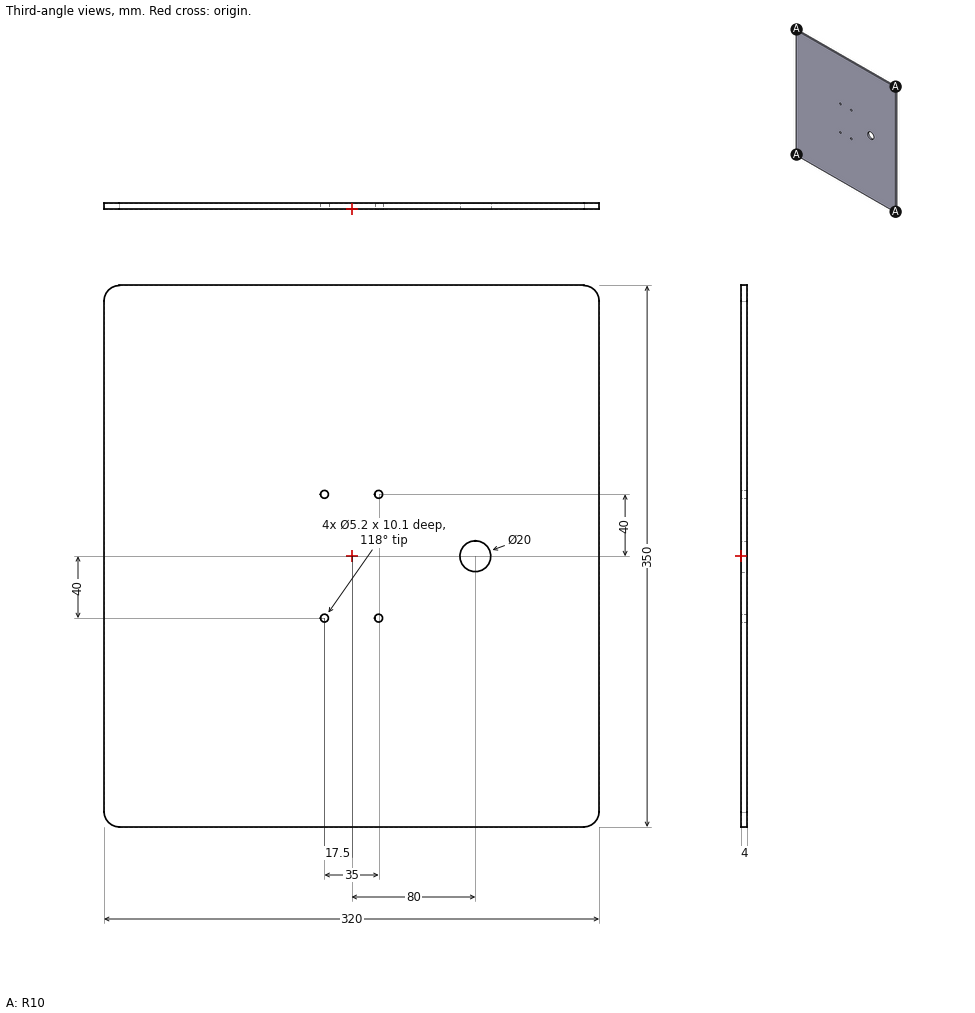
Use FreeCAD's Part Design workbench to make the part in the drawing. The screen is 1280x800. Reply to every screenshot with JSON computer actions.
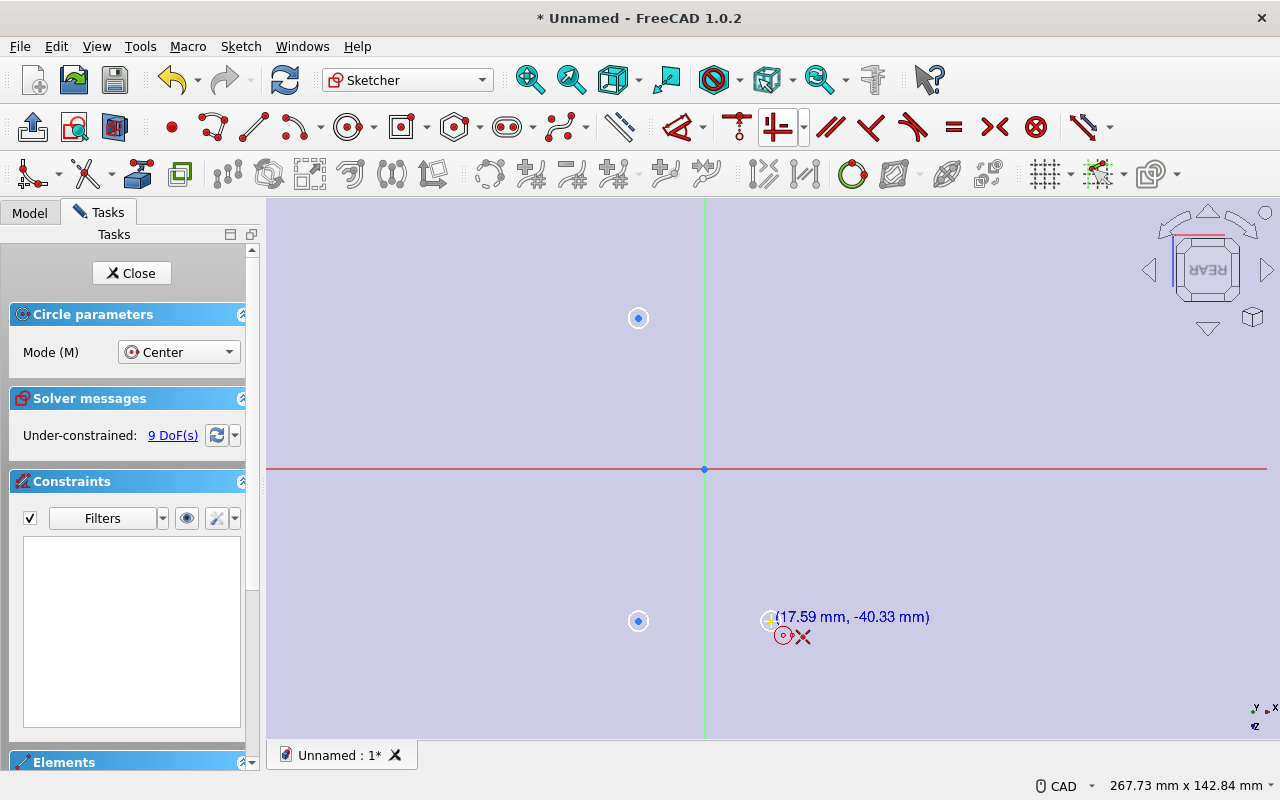
{"action": "scroll", "coordinate": [771, 318], "scroll_direction": "up", "scroll_amount": 5}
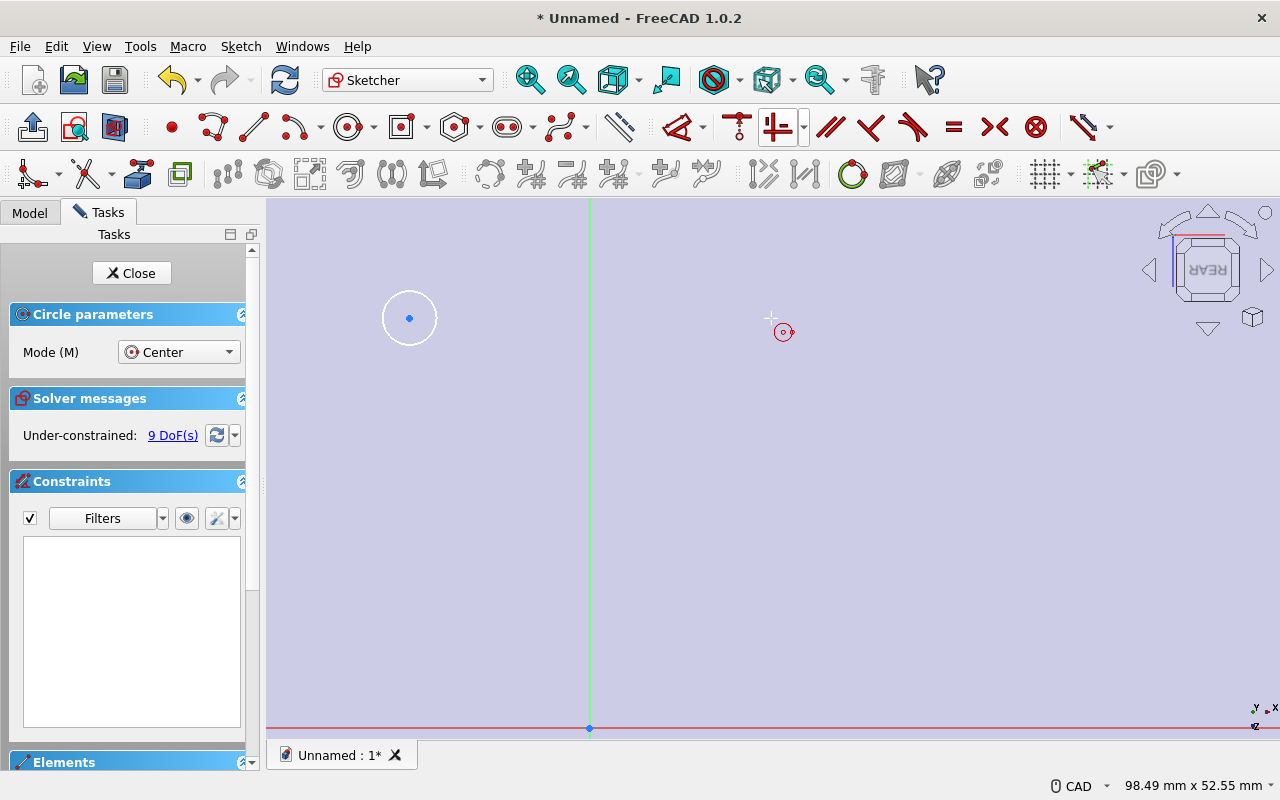
{"action": "left_click", "coordinate": [770, 317]}
{"action": "left_click", "coordinate": [789, 298]}
{"action": "key", "text": "Escape"}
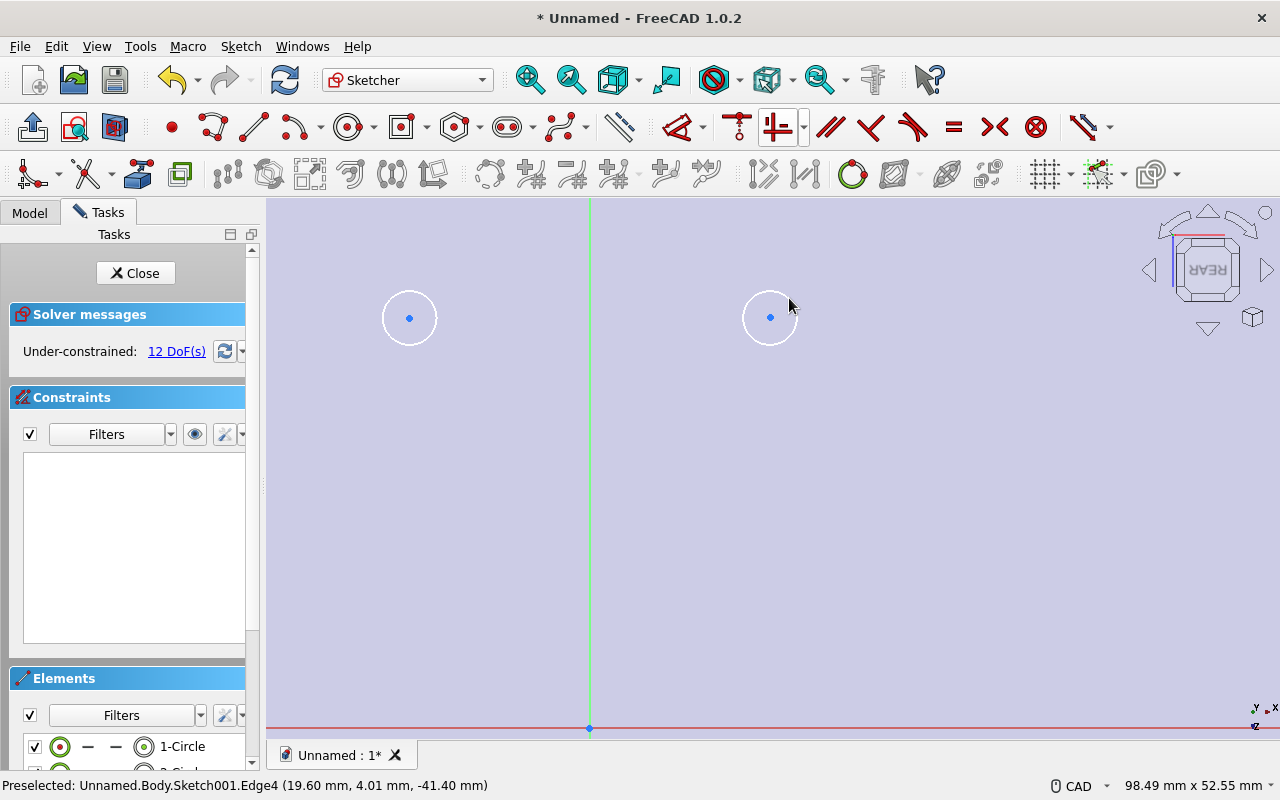
{"action": "left_click", "coordinate": [429, 299]}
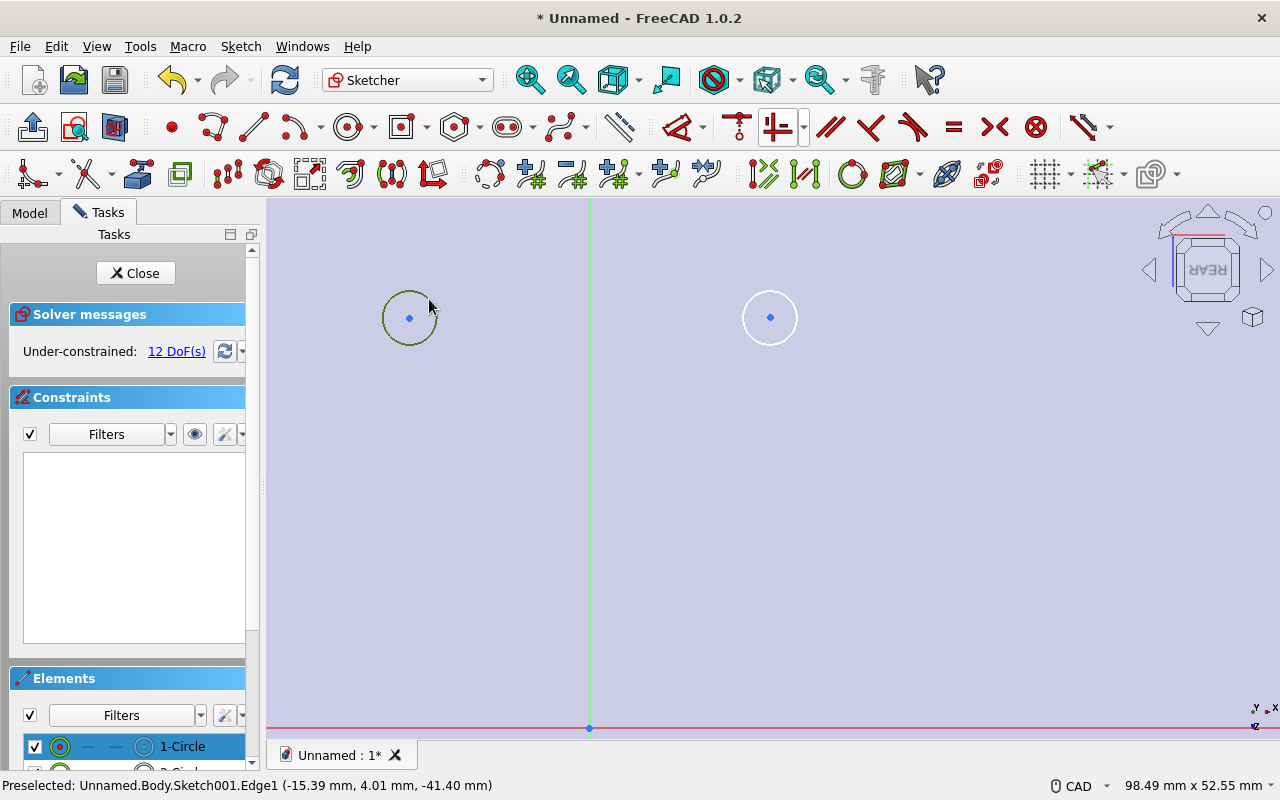
{"action": "scroll", "coordinate": [771, 317], "scroll_direction": "down", "scroll_amount": 5}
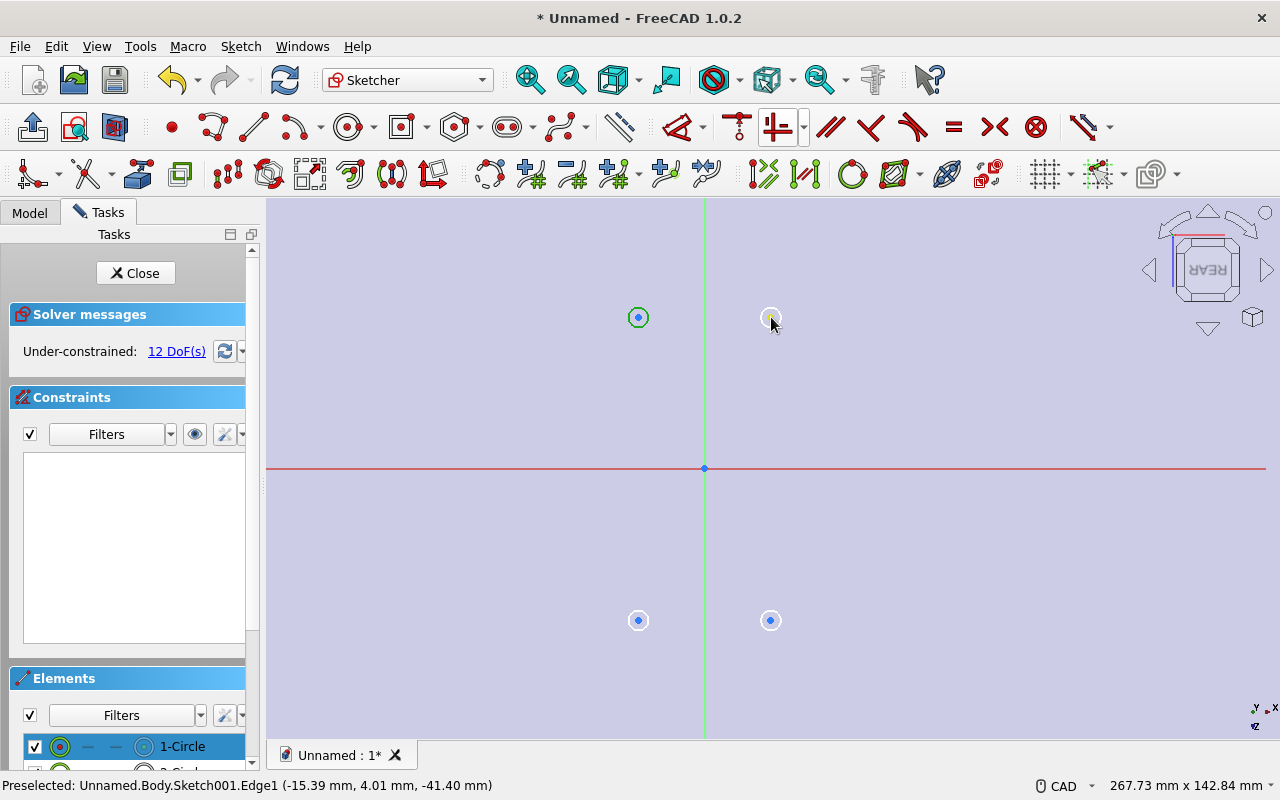
{"action": "scroll", "coordinate": [778, 613], "scroll_direction": "up", "scroll_amount": 2}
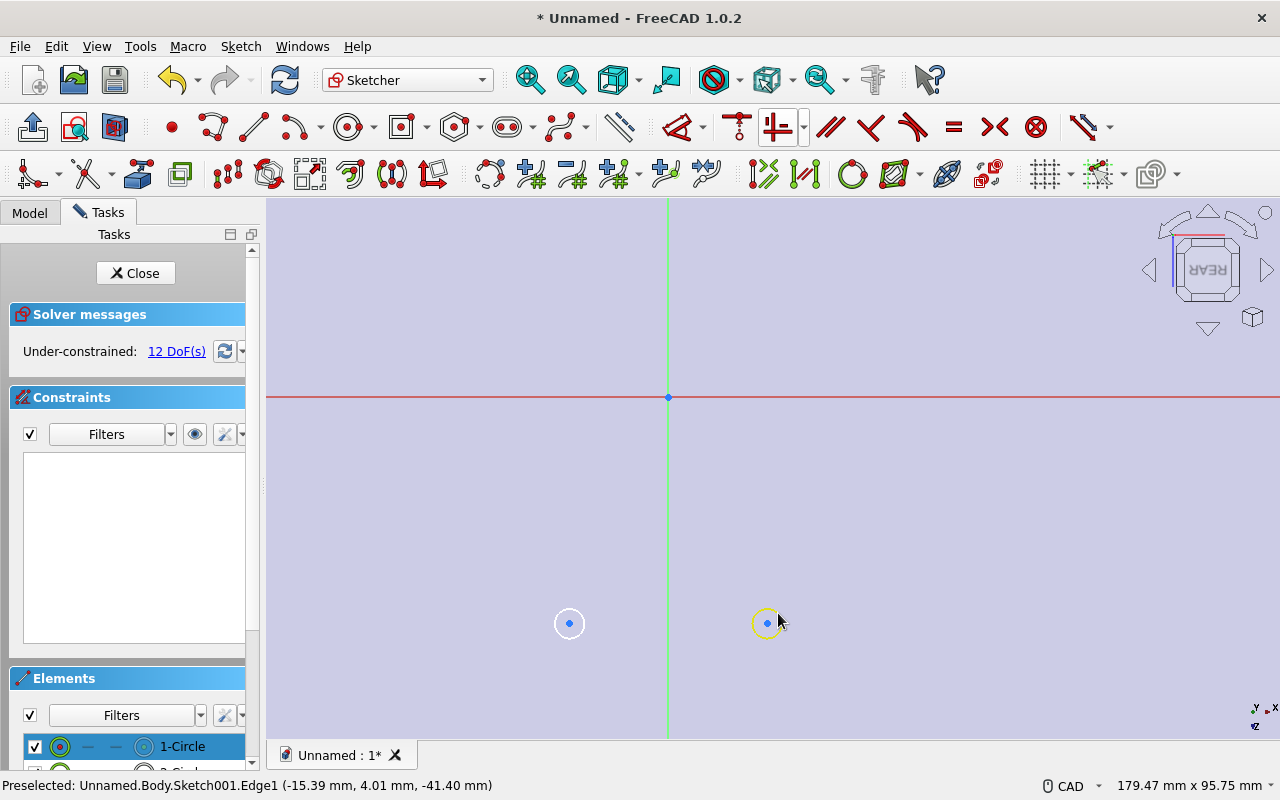
{"action": "left_click", "coordinate": [778, 613]}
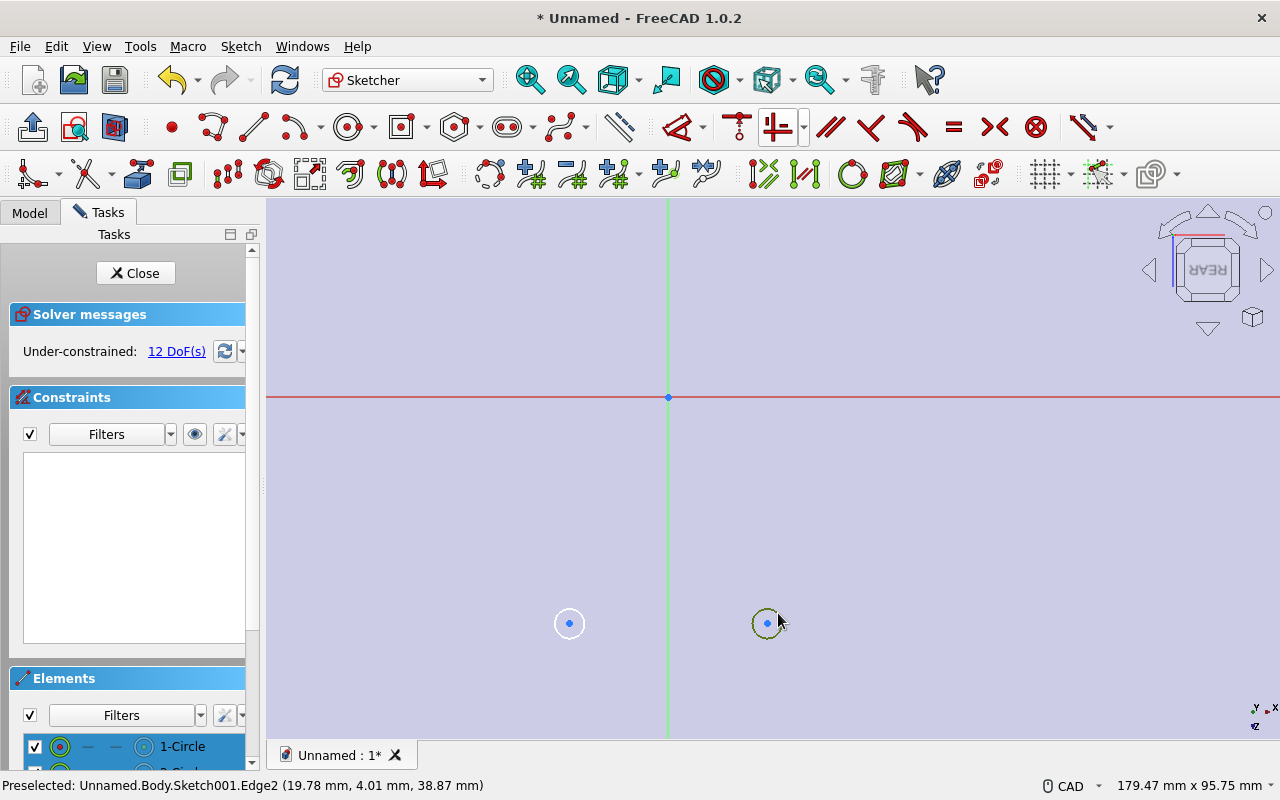
{"action": "left_click", "coordinate": [580, 613]}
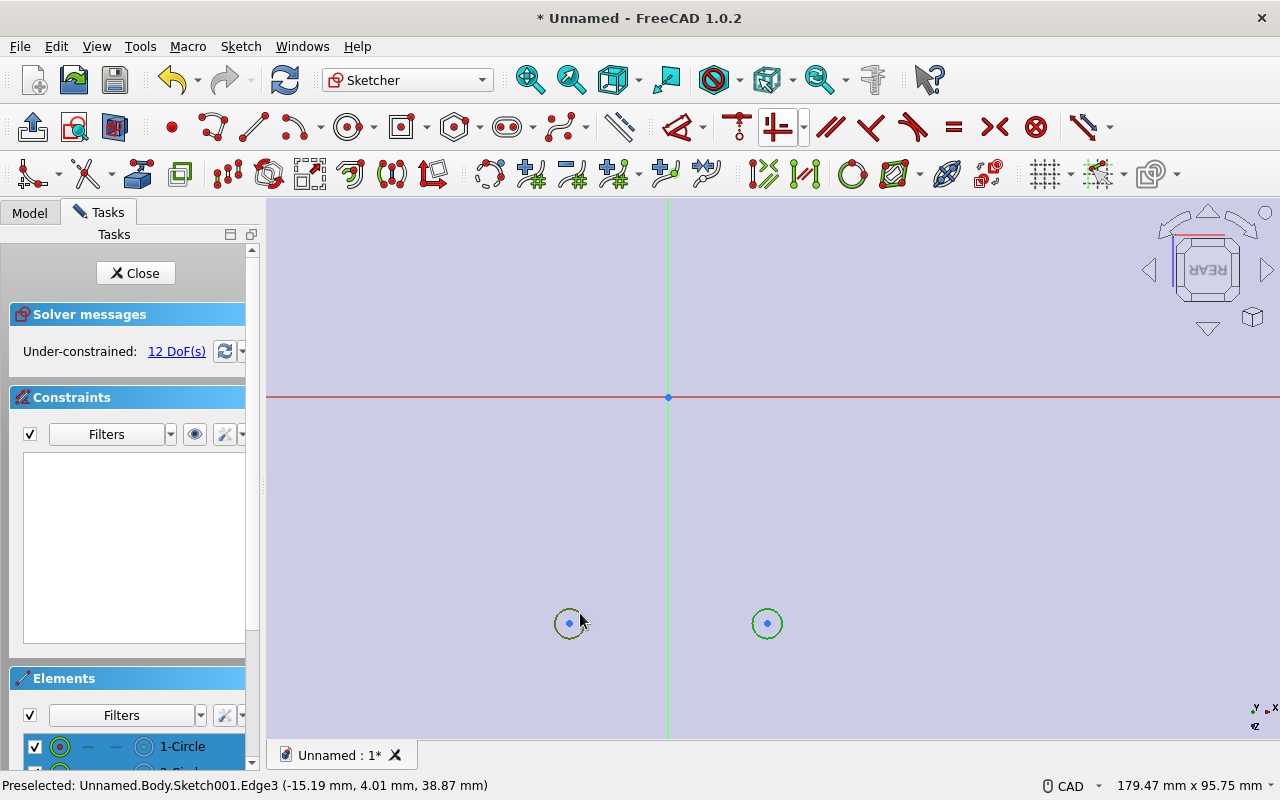
{"action": "scroll", "coordinate": [778, 614], "scroll_direction": "down", "scroll_amount": 2}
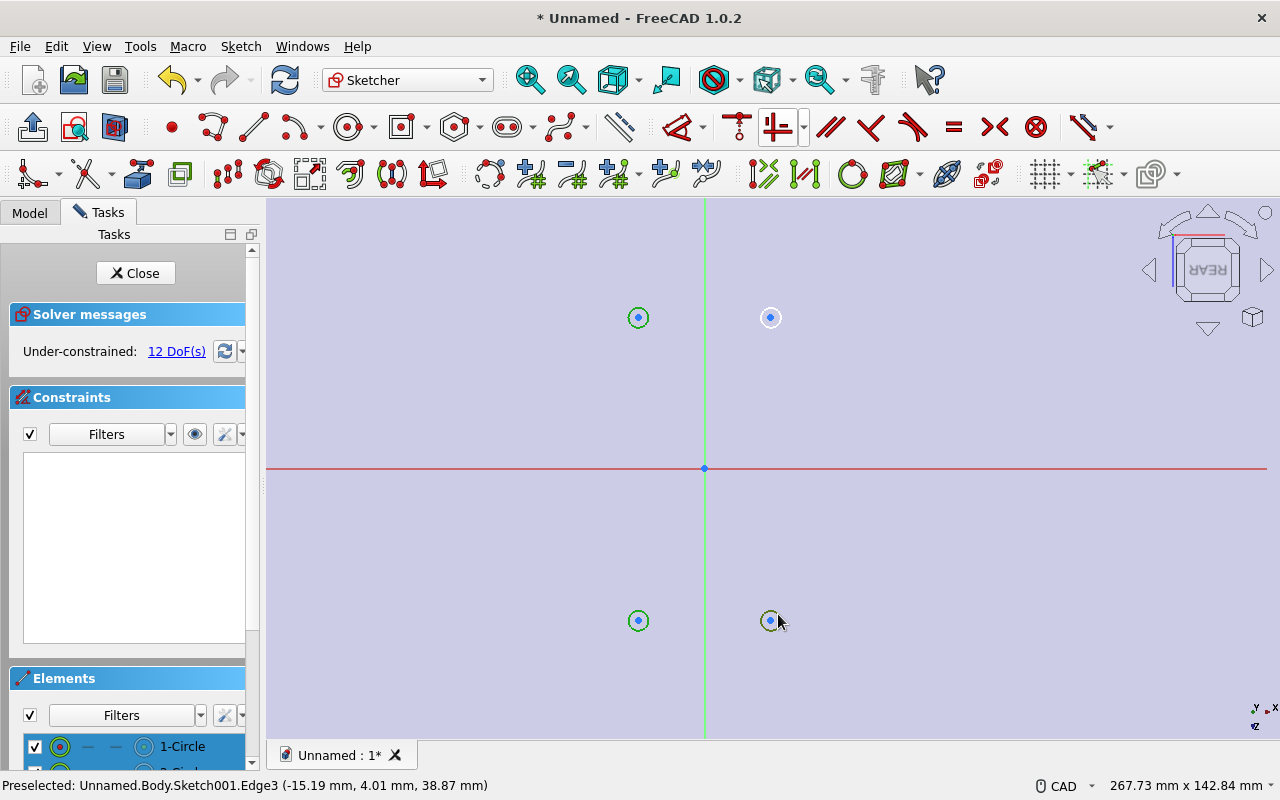
{"action": "scroll", "coordinate": [778, 311], "scroll_direction": "up", "scroll_amount": 2}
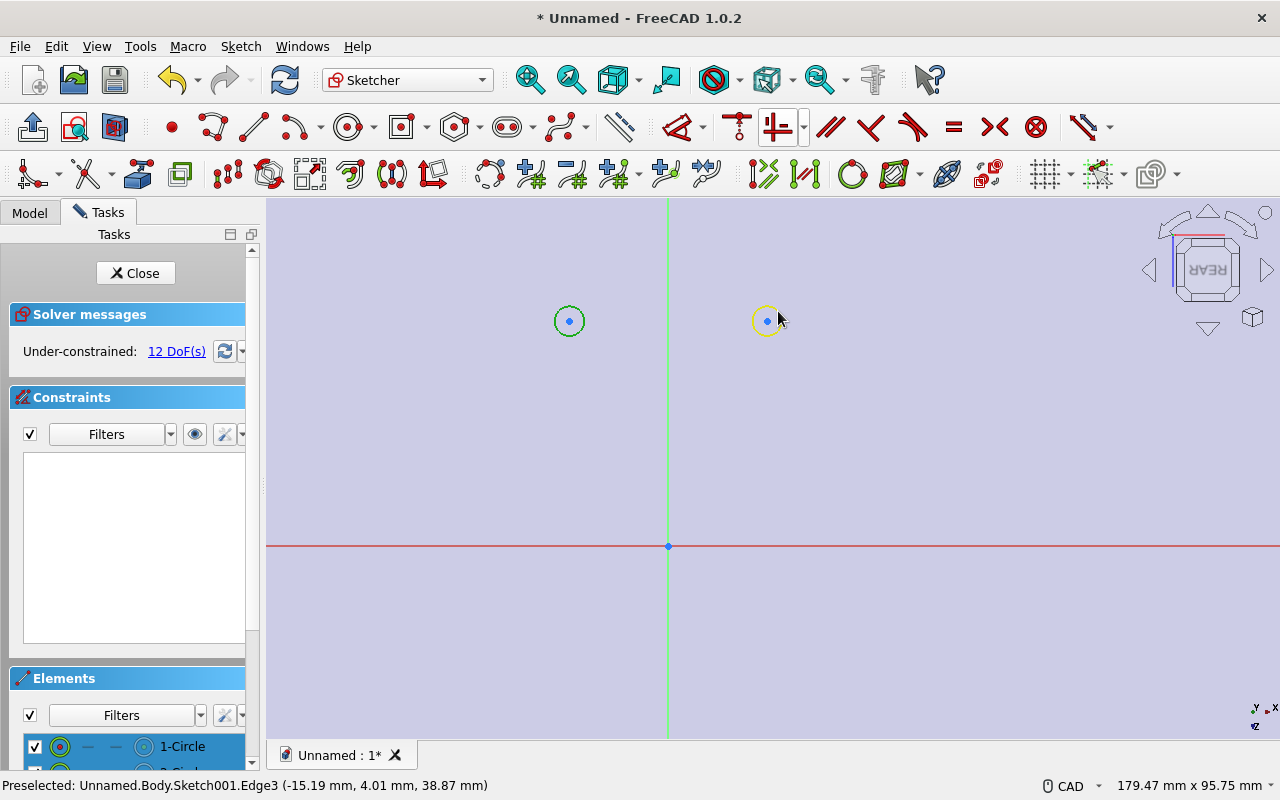
{"action": "left_click", "coordinate": [778, 311]}